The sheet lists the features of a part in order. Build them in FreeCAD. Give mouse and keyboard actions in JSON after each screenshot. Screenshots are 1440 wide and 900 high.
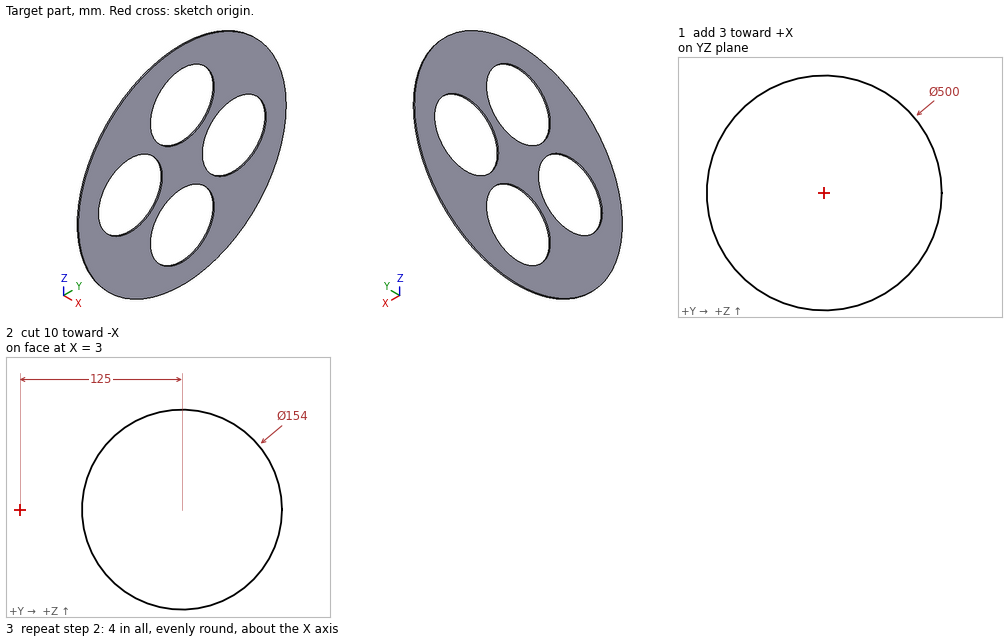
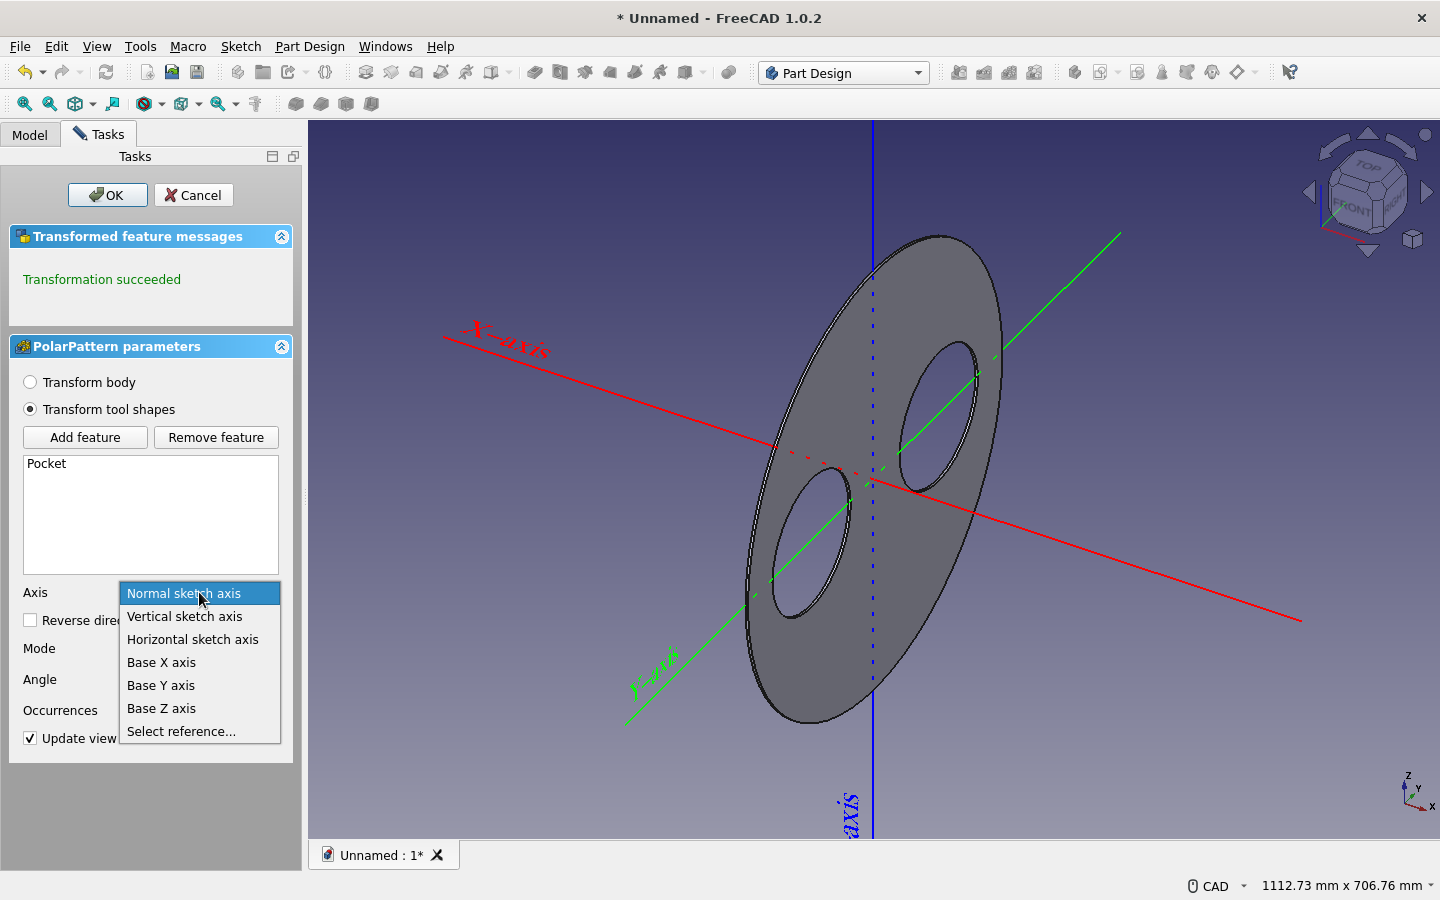
{"action": "left_click", "coordinate": [198, 662]}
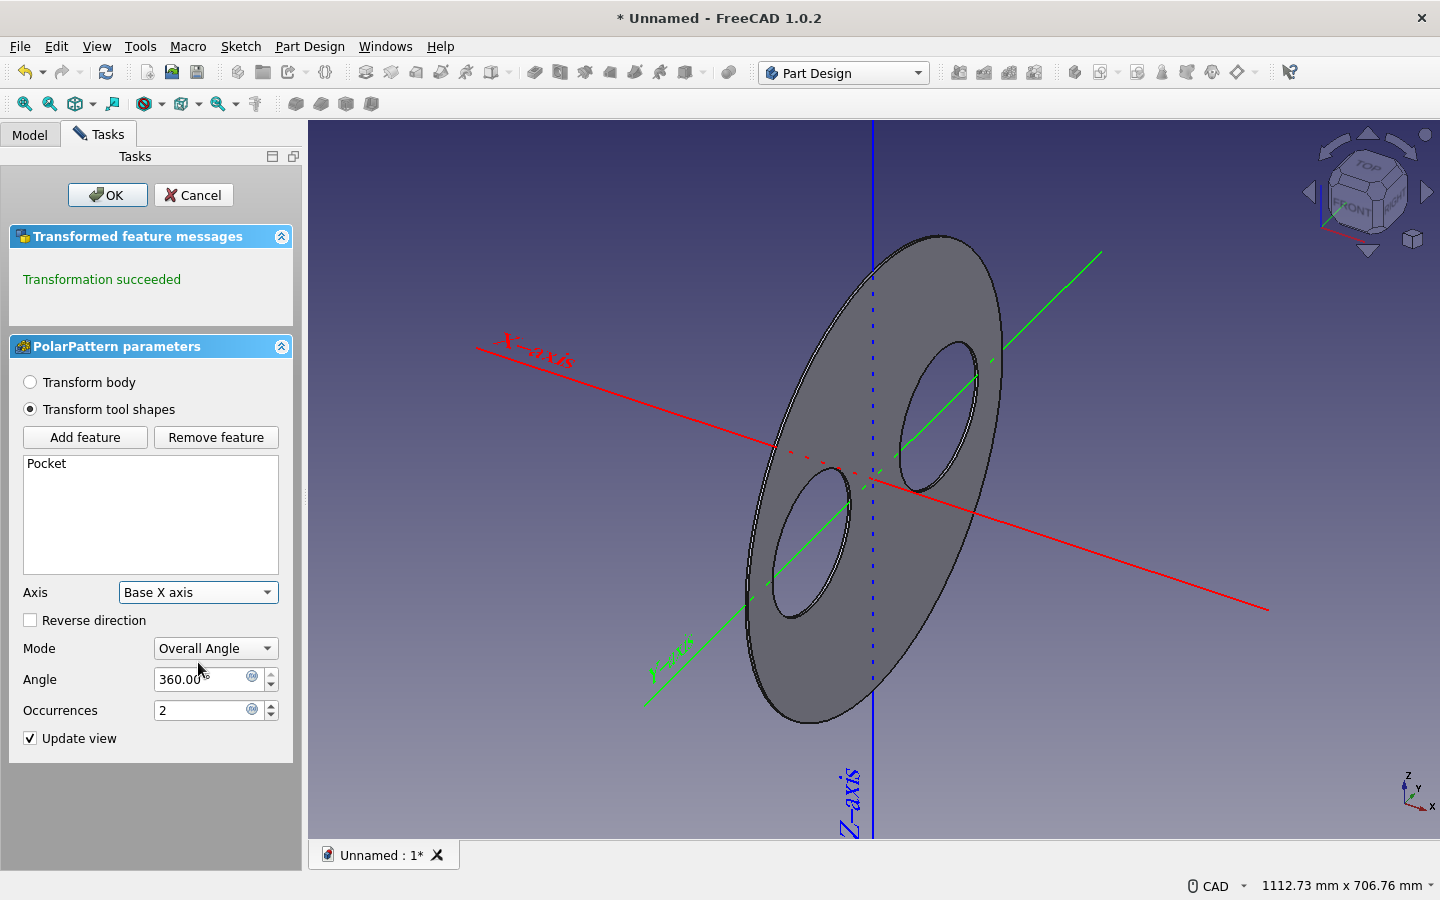
{"action": "triple_click", "coordinate": [210, 710]}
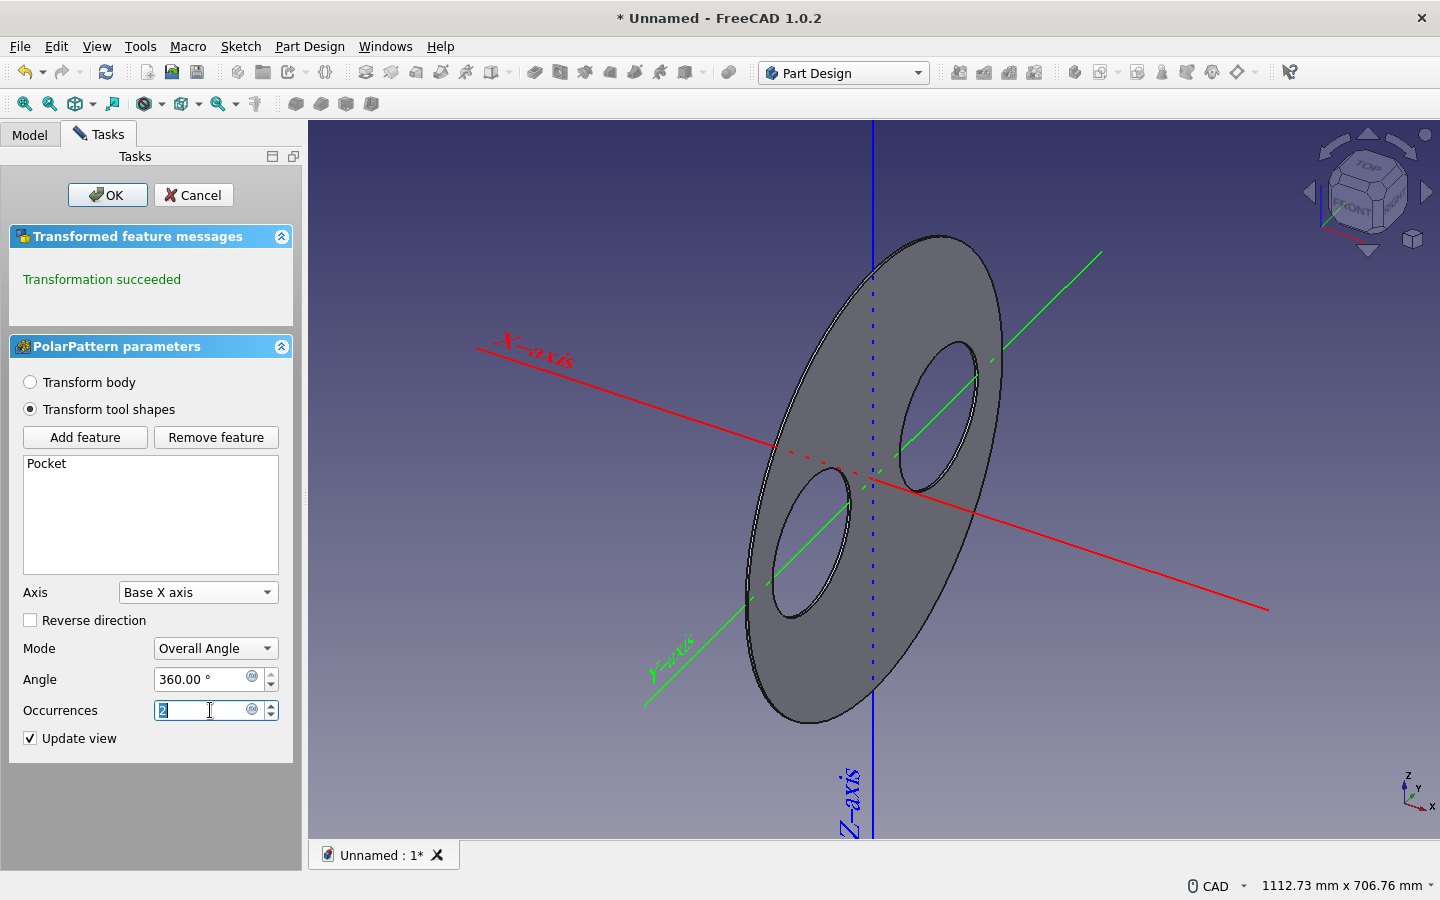
{"action": "type", "text": "4"}
{"action": "key", "text": "Tab"}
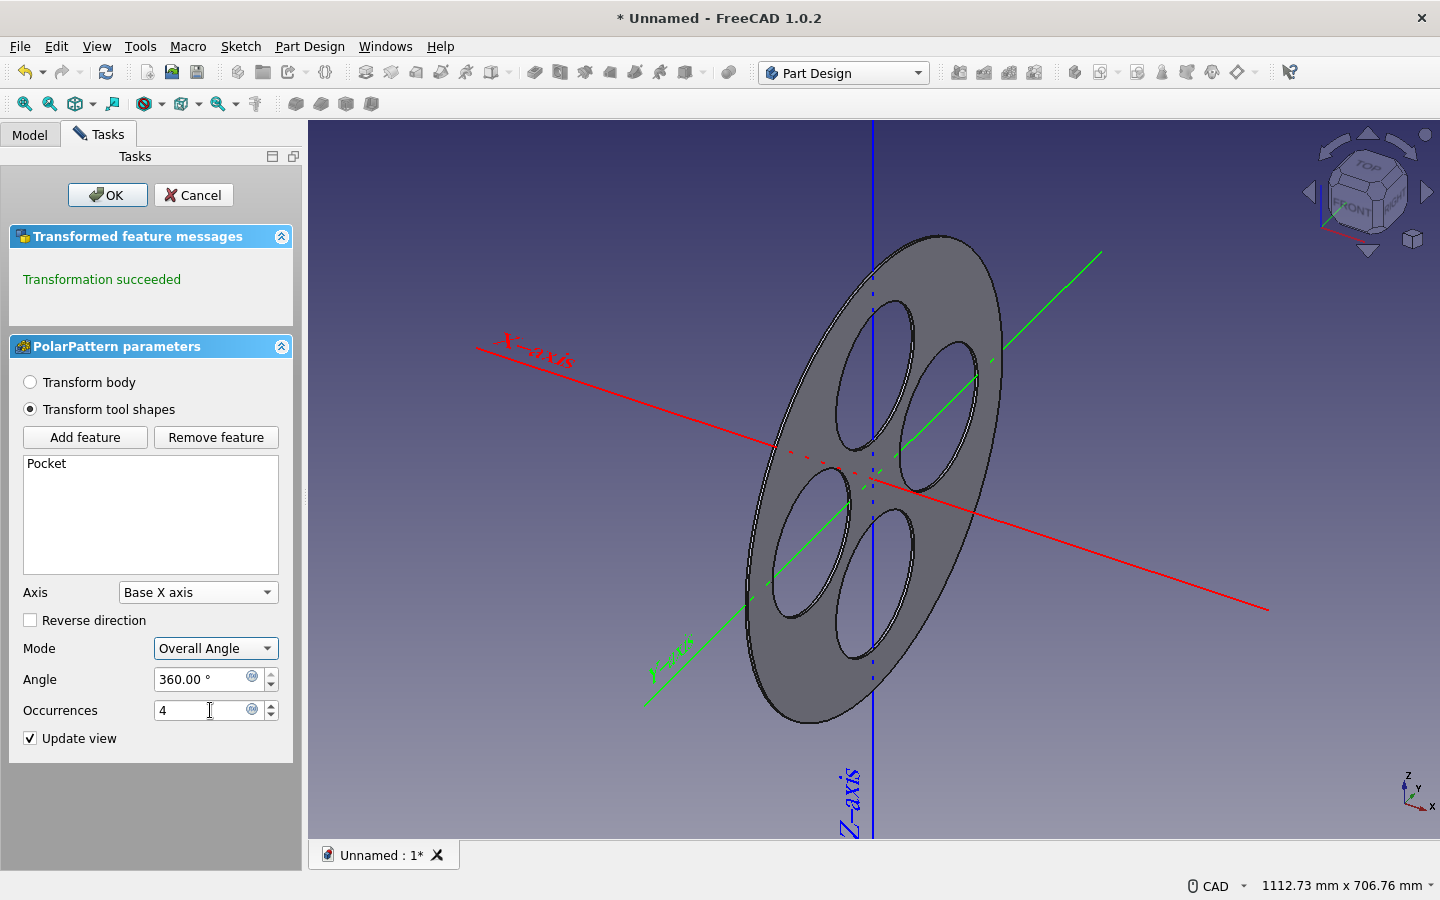
{"action": "left_click", "coordinate": [108, 195]}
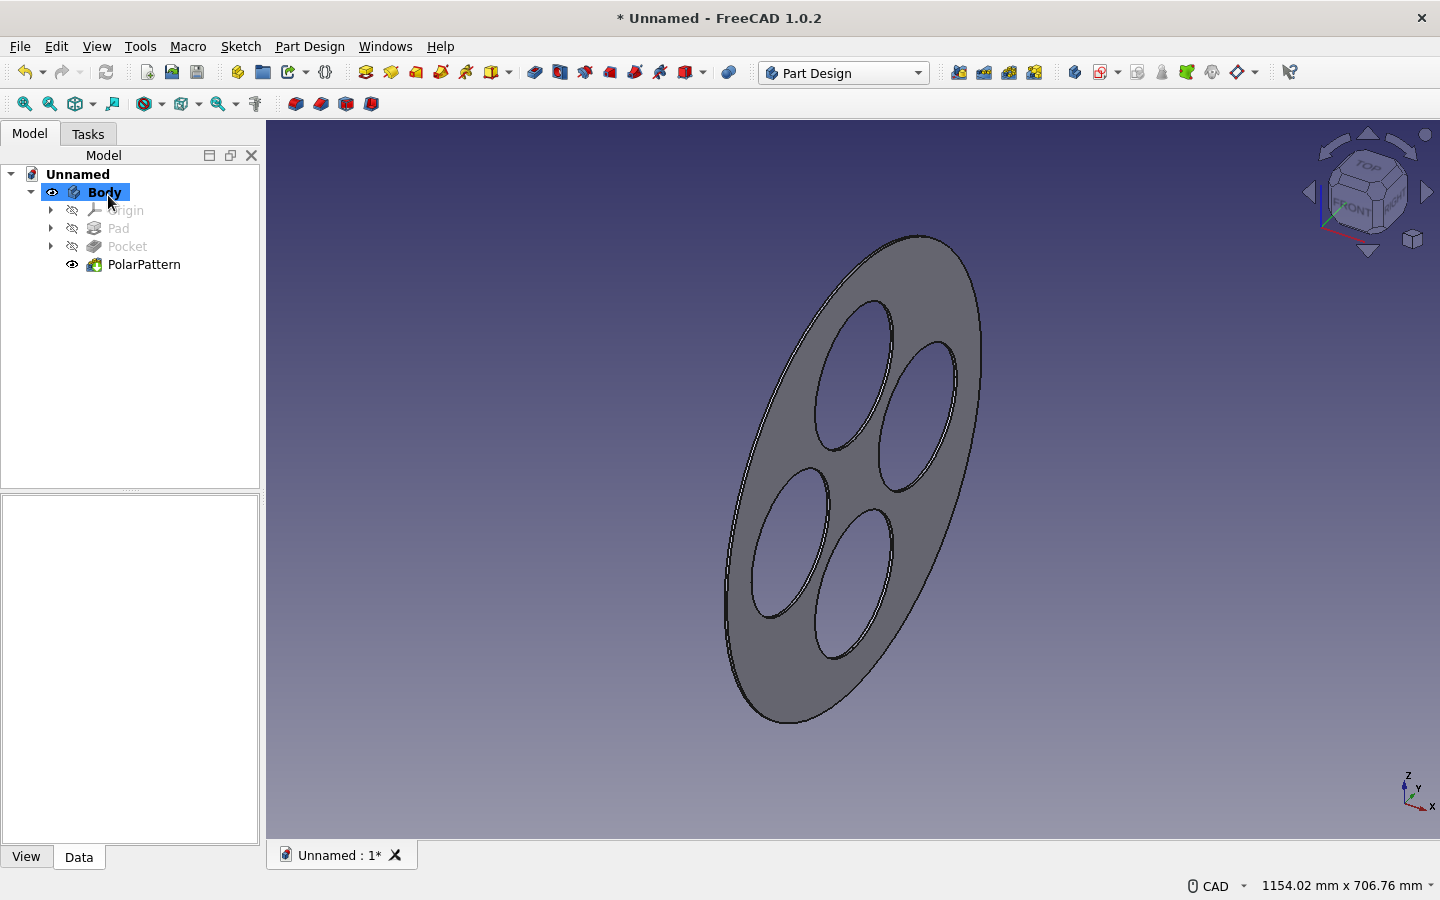
{"action": "key", "text": "0"}